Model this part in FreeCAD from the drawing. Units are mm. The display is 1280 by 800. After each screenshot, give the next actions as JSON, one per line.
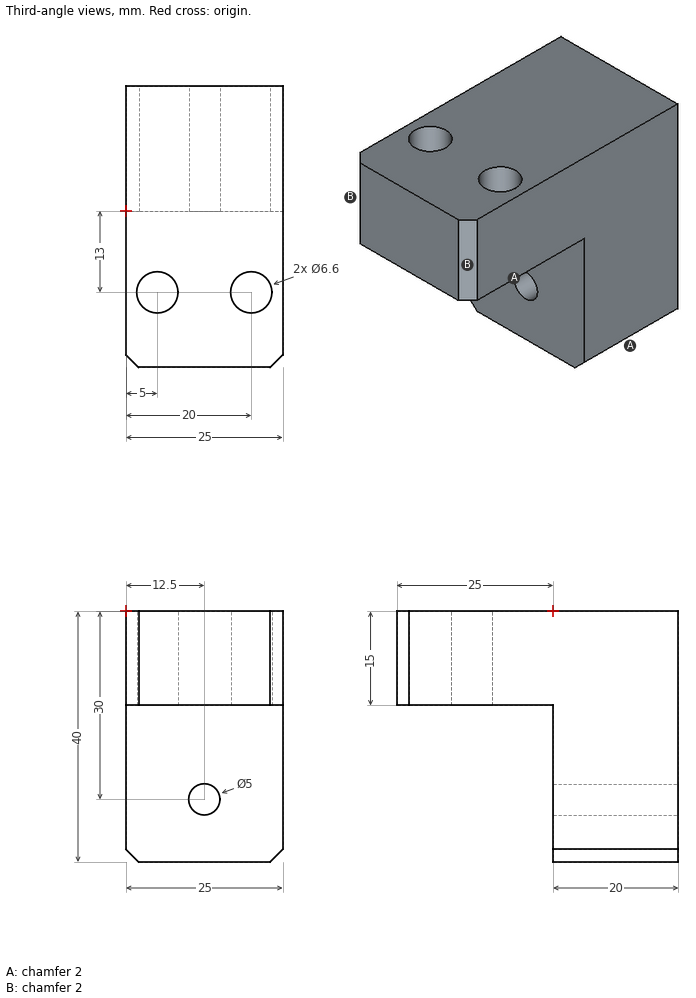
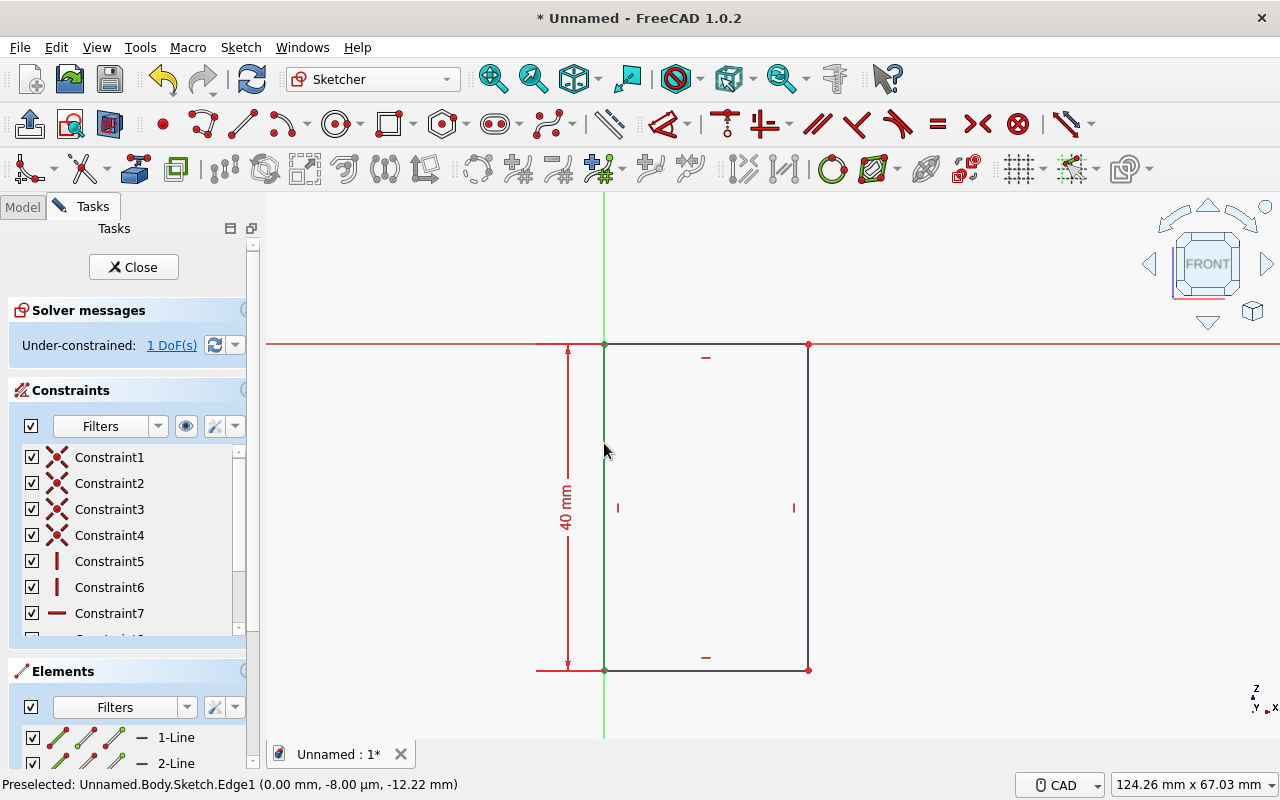
{"action": "left_click", "coordinate": [665, 671]}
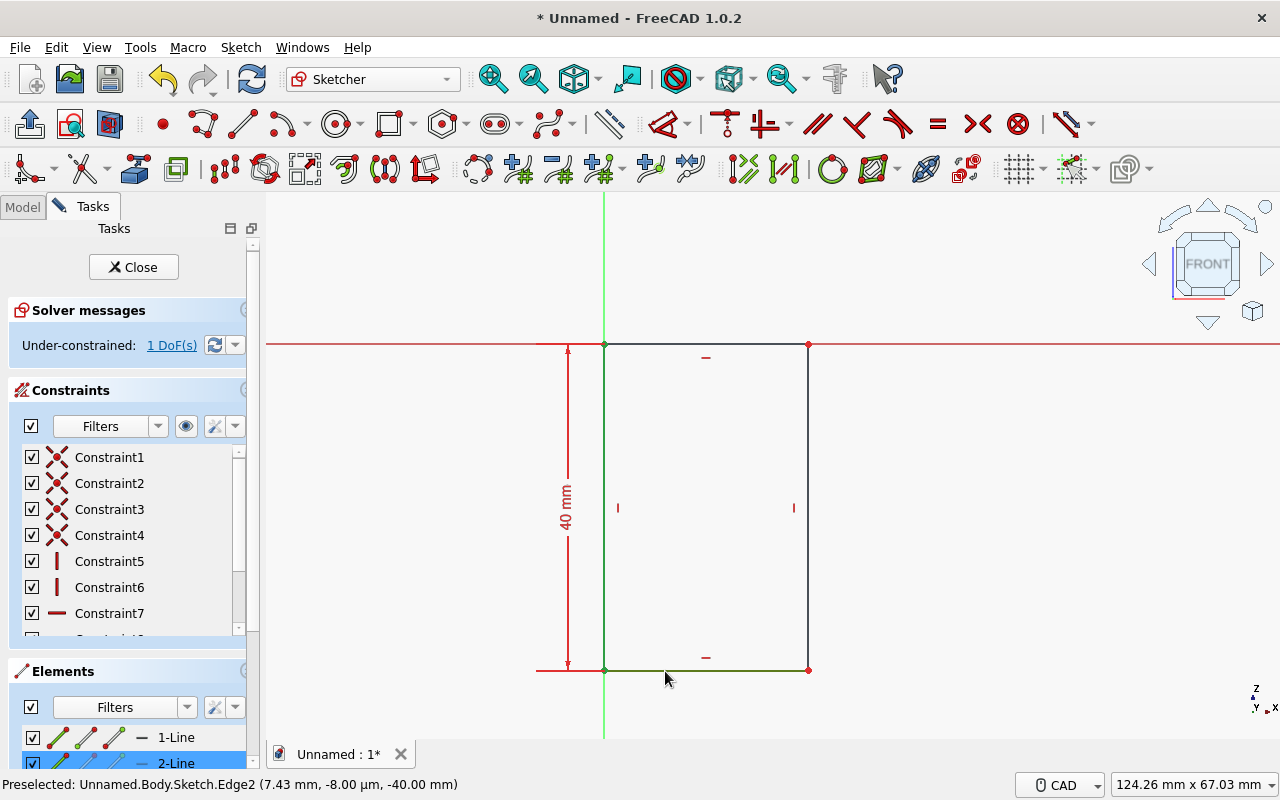
{"action": "key", "text": "l"}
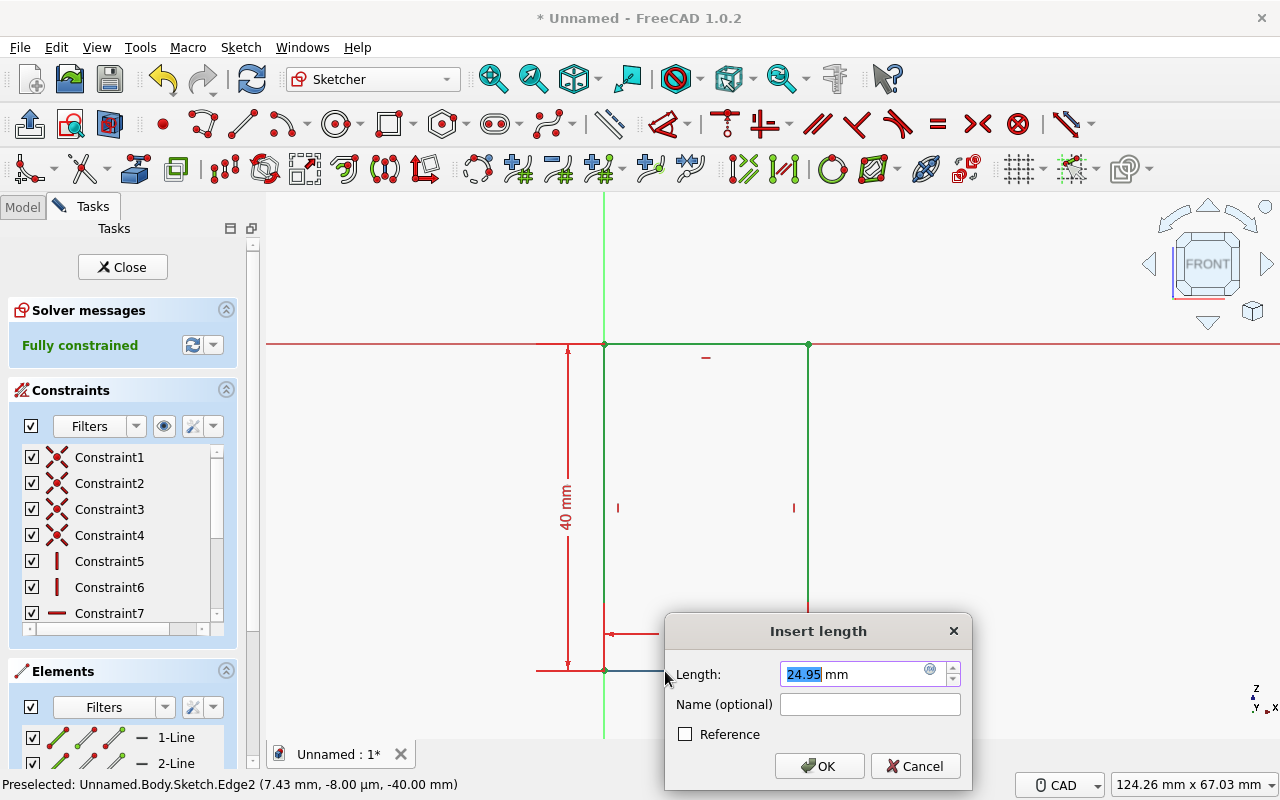
{"action": "type", "text": "25"}
{"action": "key", "text": "Return"}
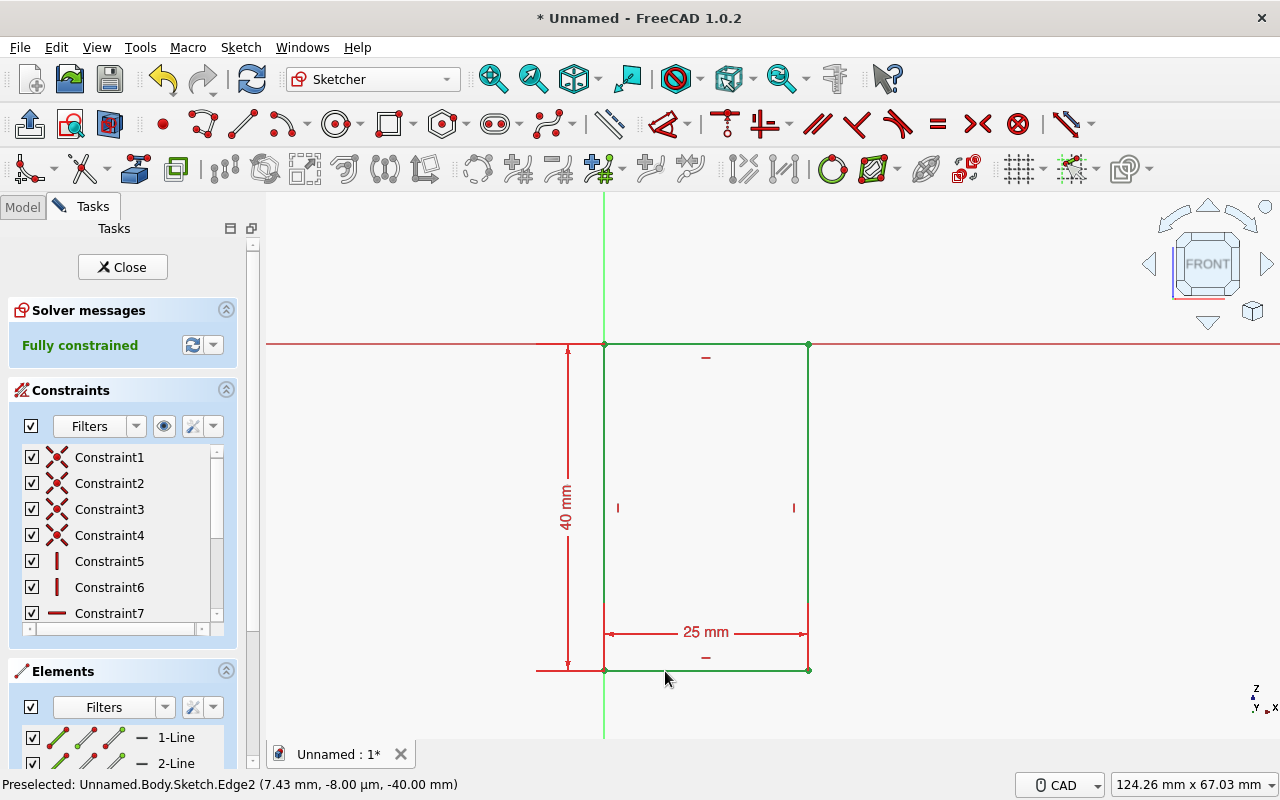
{"action": "left_click", "coordinate": [123, 267]}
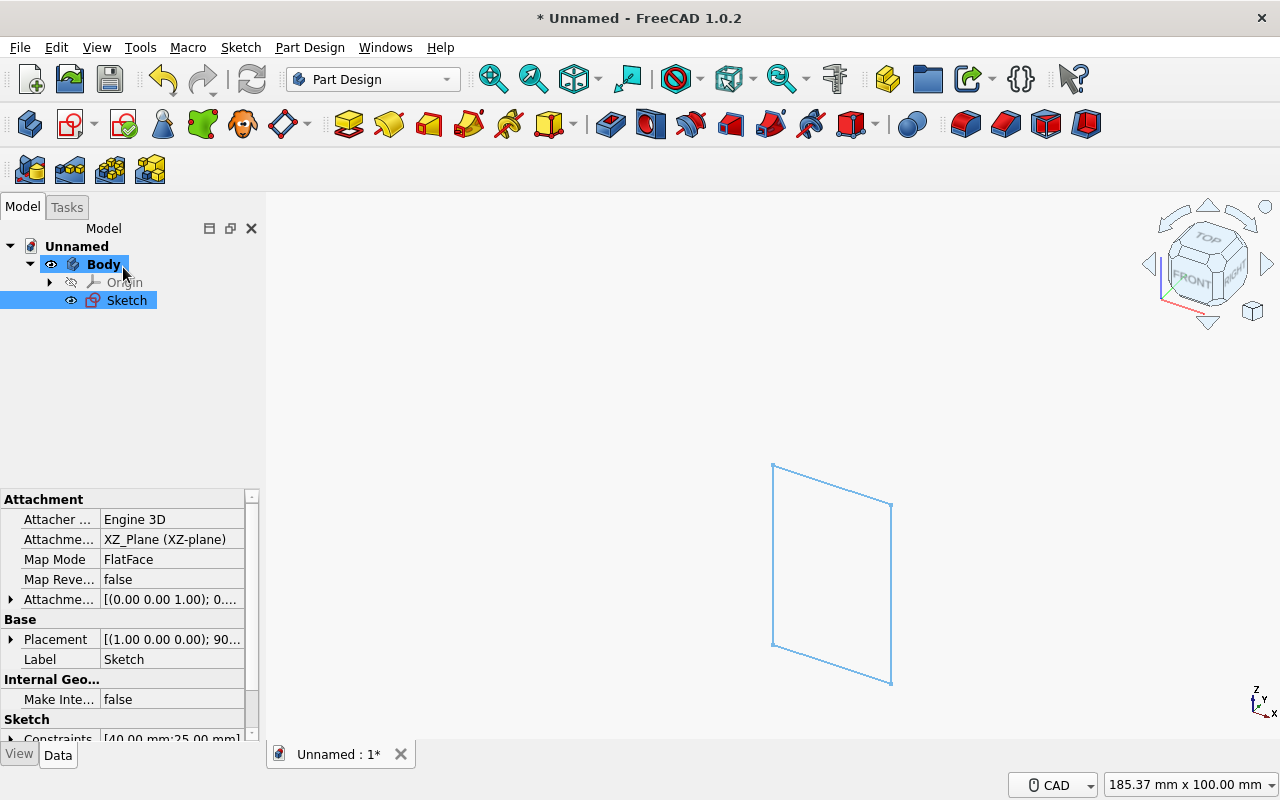
{"action": "left_click", "coordinate": [350, 124]}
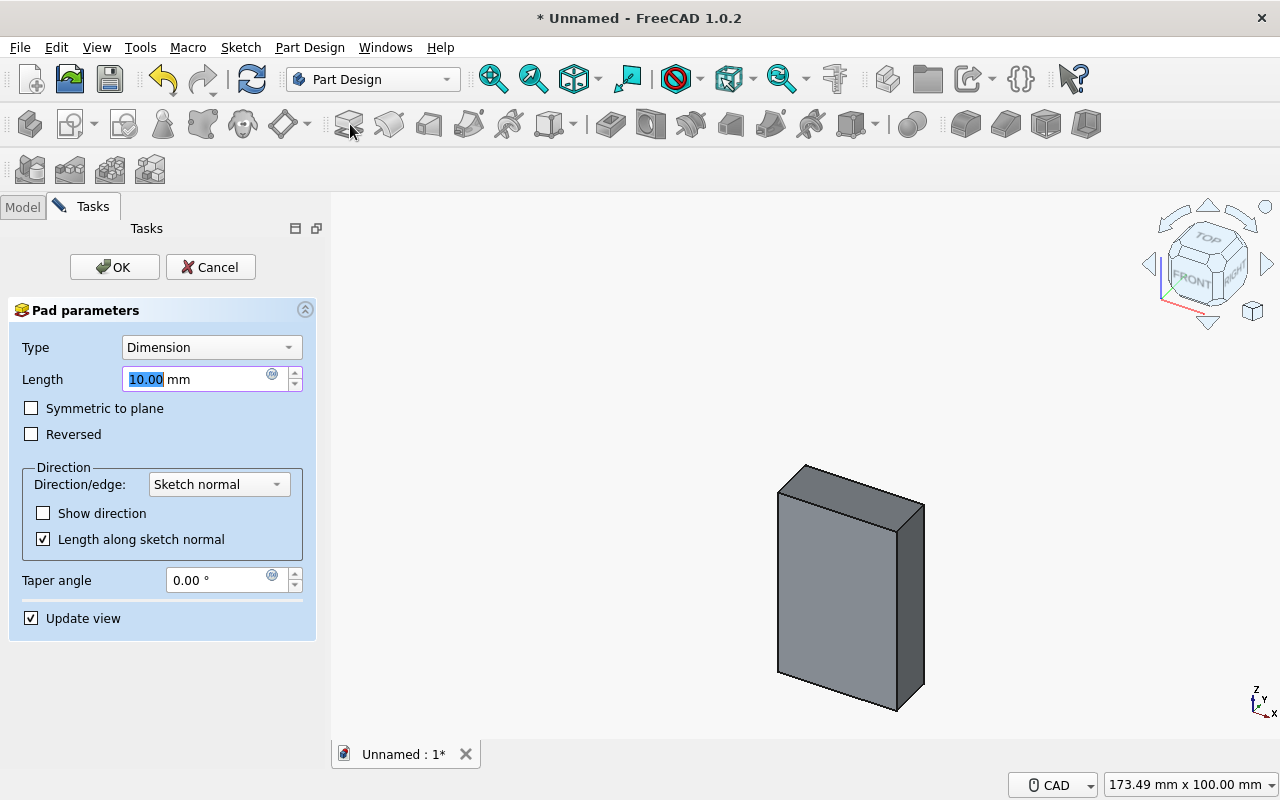
{"action": "type", "text": "20"}
{"action": "key", "text": "Tab"}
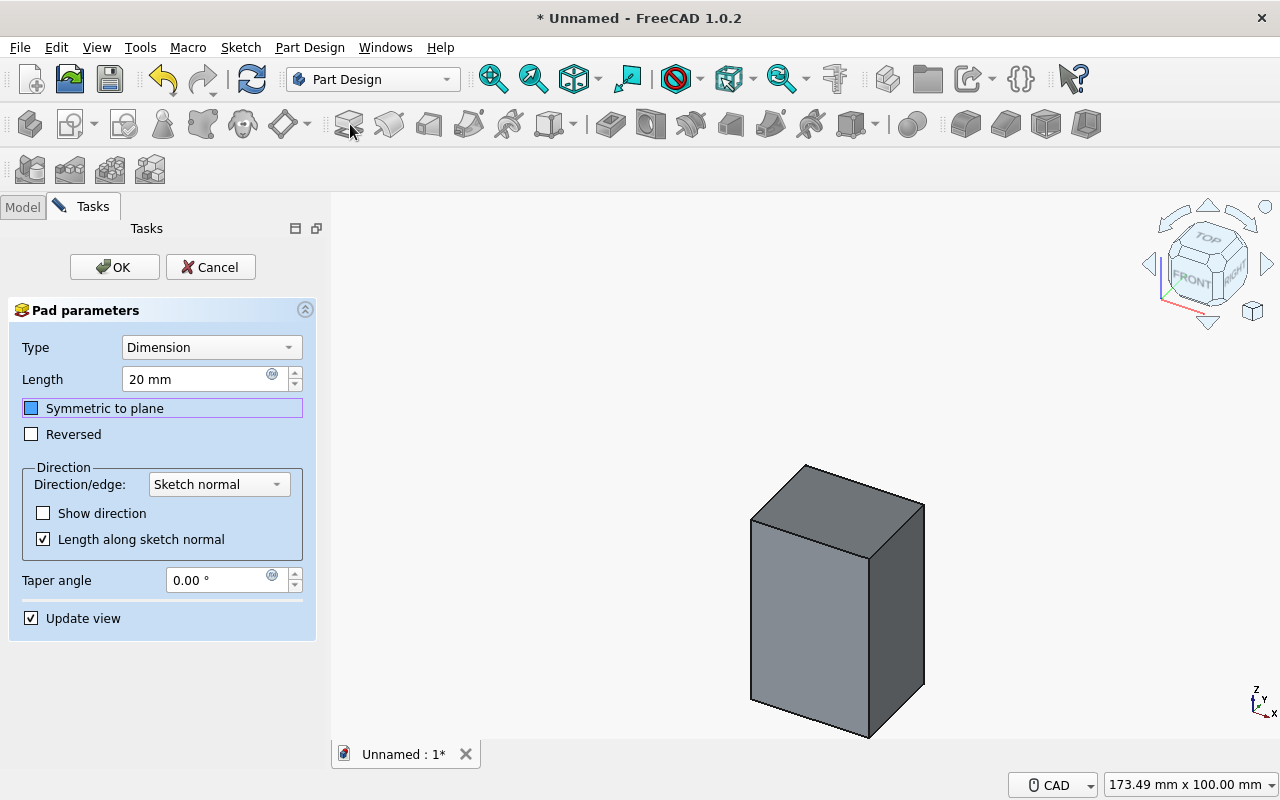
{"action": "left_click", "coordinate": [30, 434]}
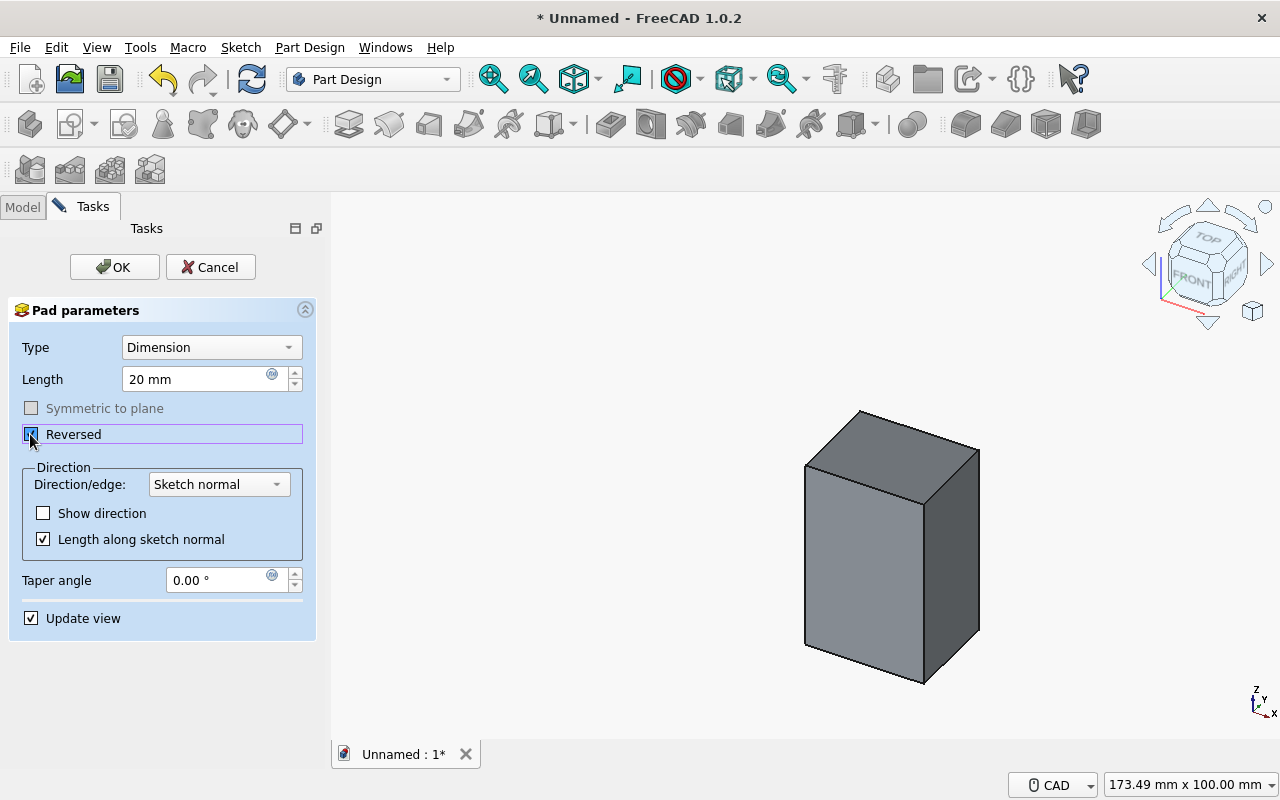
{"action": "left_click", "coordinate": [115, 267]}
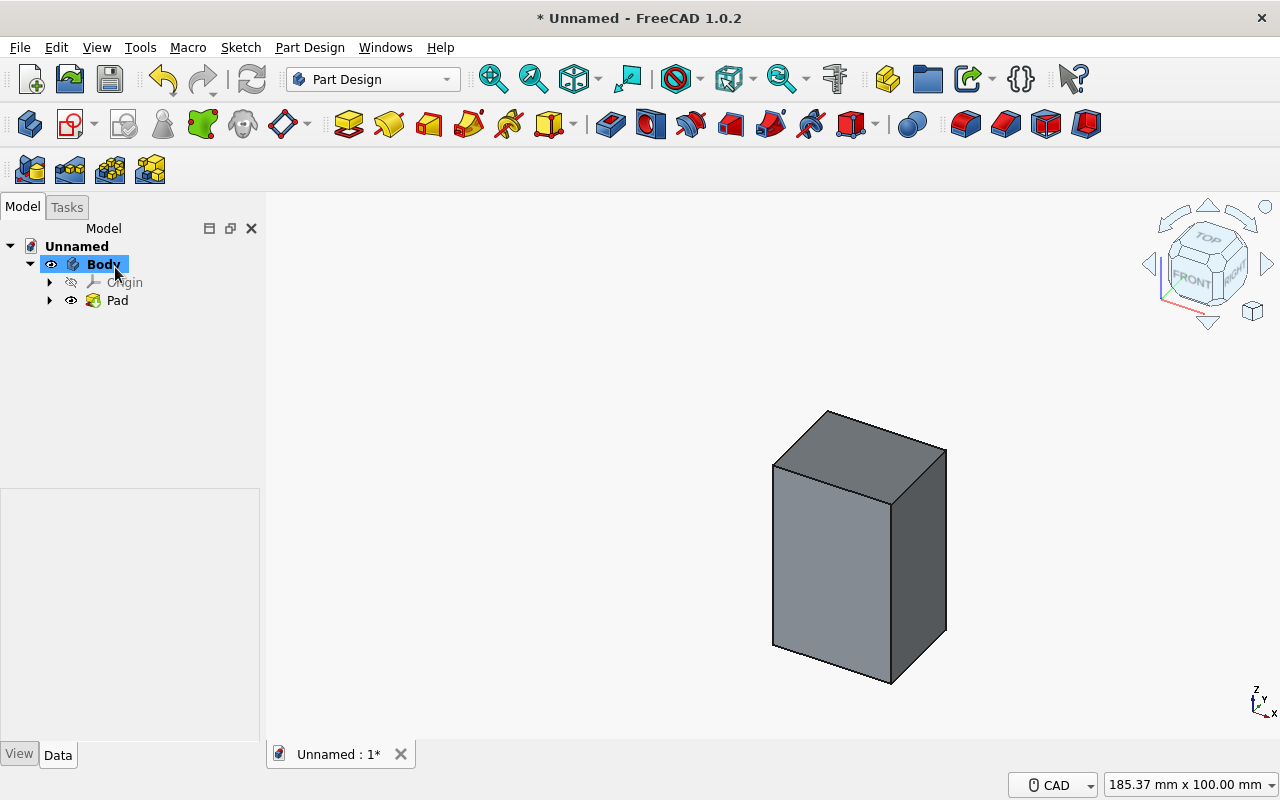
{"action": "key", "text": "0"}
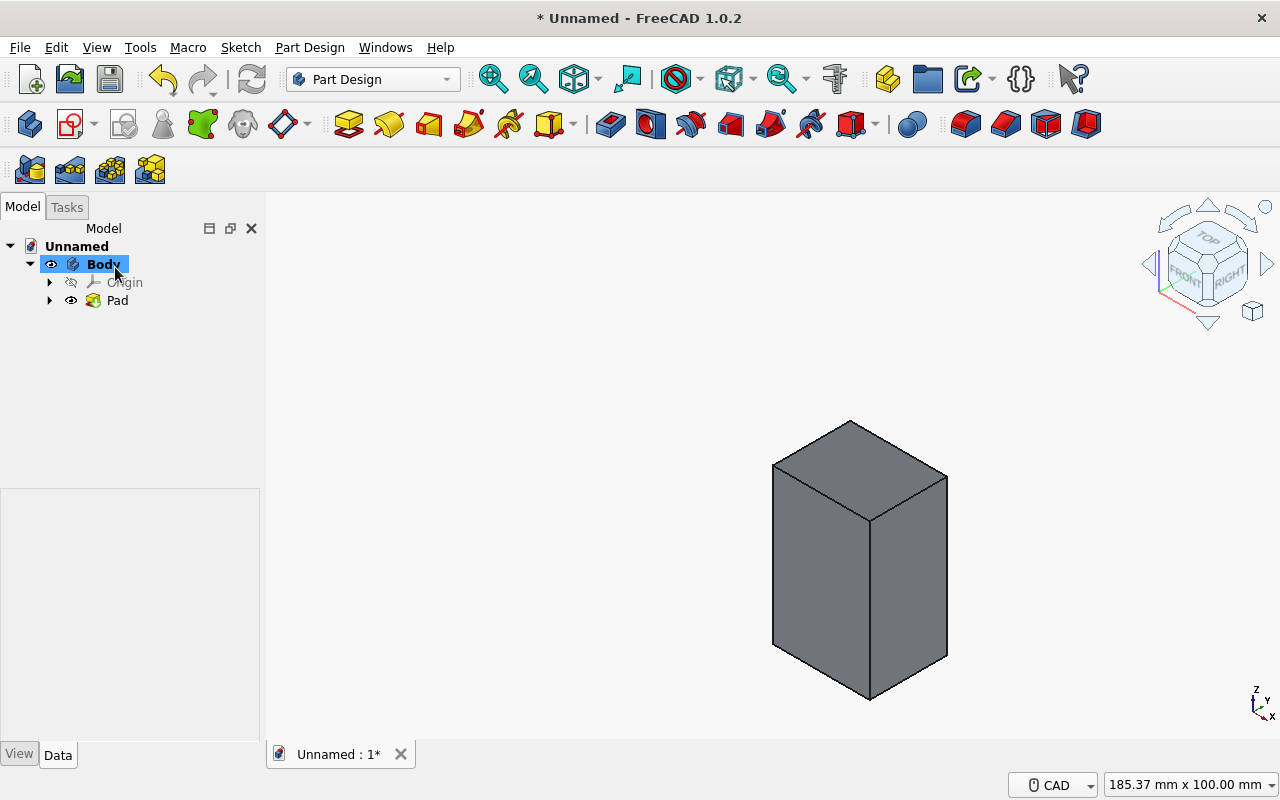
{"action": "key", "text": "2"}